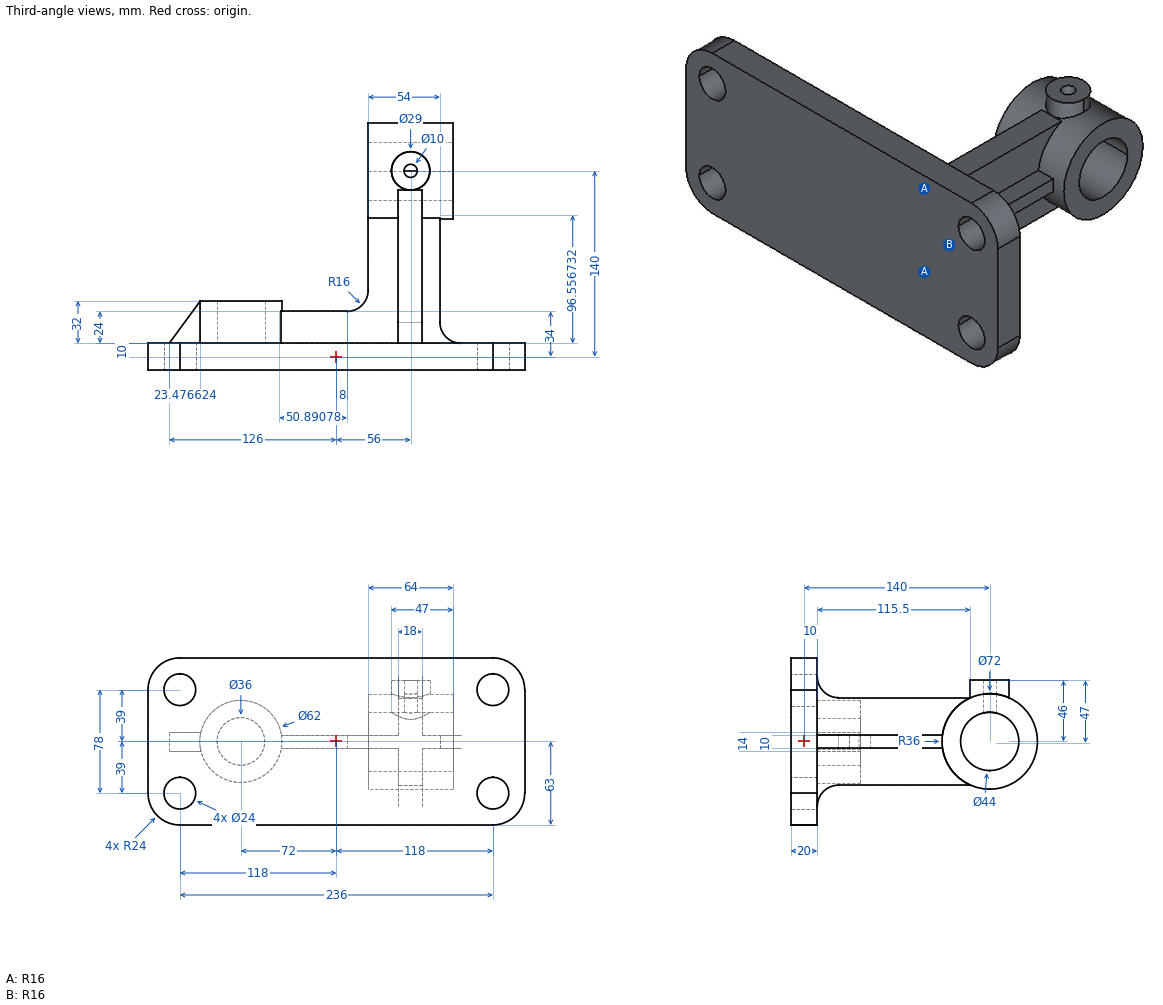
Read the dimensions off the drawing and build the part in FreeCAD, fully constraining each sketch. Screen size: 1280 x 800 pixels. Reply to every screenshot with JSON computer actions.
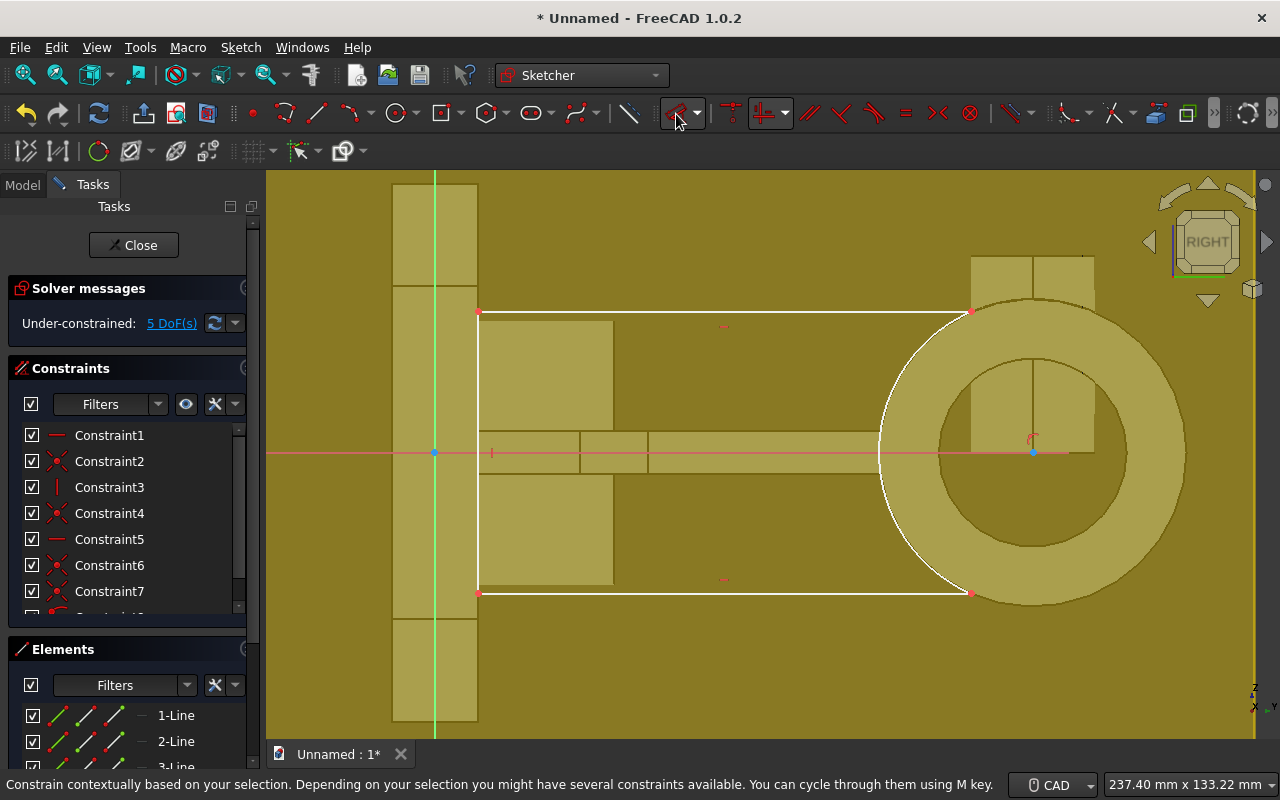
{"action": "left_click", "coordinate": [895, 384]}
{"action": "left_click", "coordinate": [866, 370]}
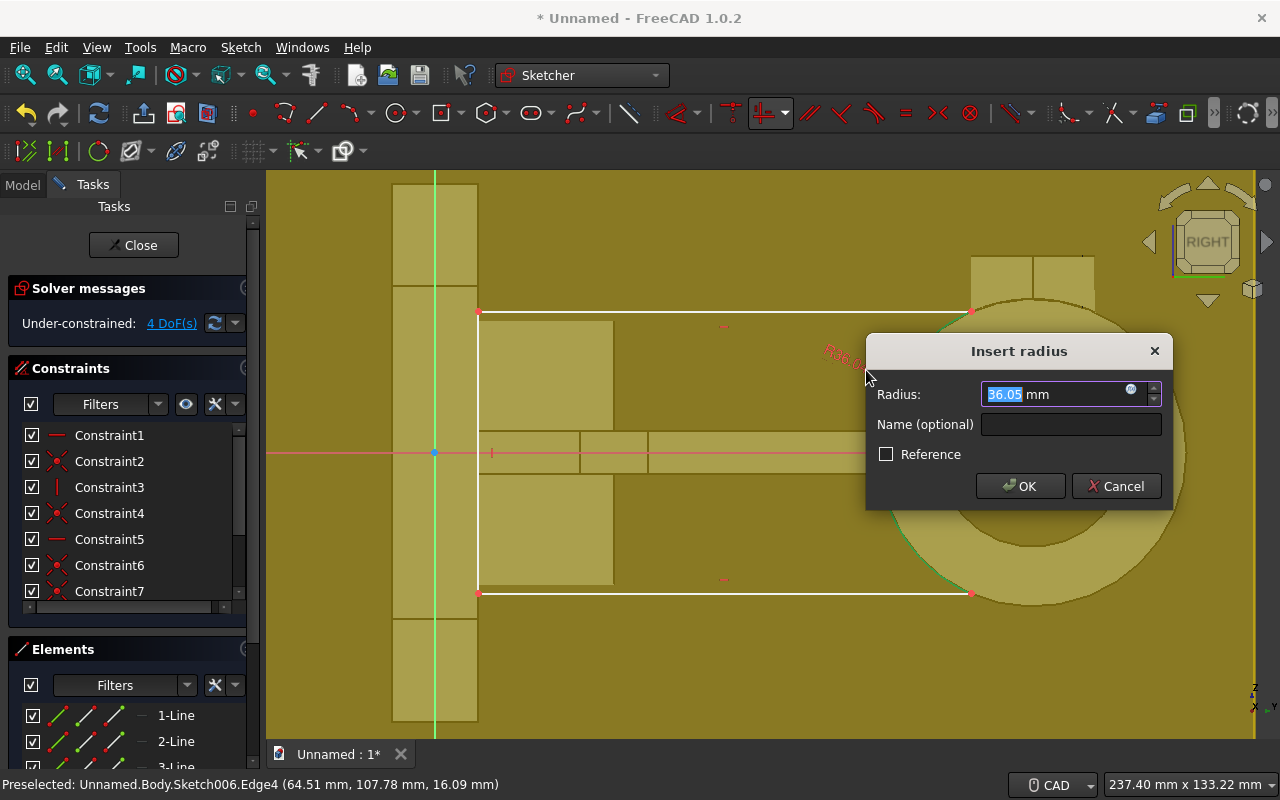
{"action": "type", "text": "36"}
{"action": "key", "text": "Return"}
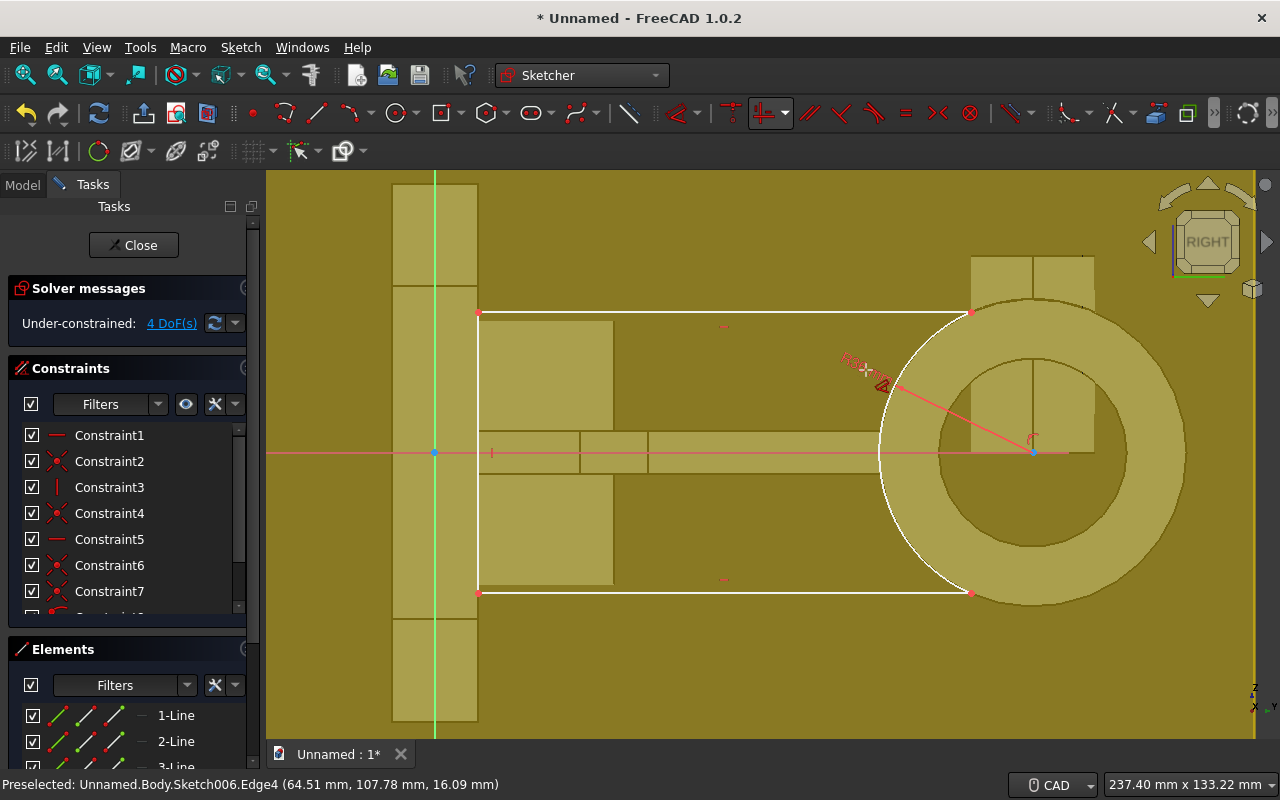
{"action": "left_click", "coordinate": [478, 312]}
{"action": "left_click", "coordinate": [456, 278]}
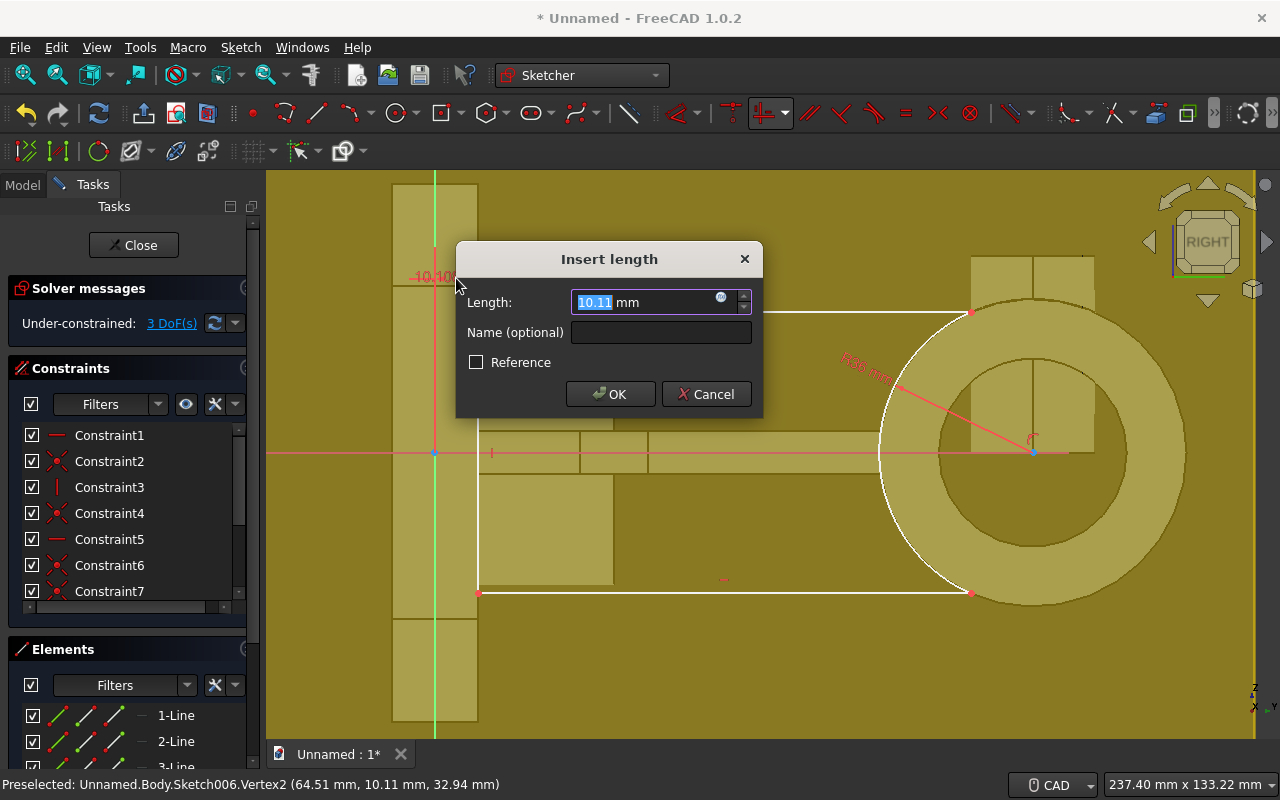
{"action": "type", "text": "10"}
{"action": "key", "text": "Return"}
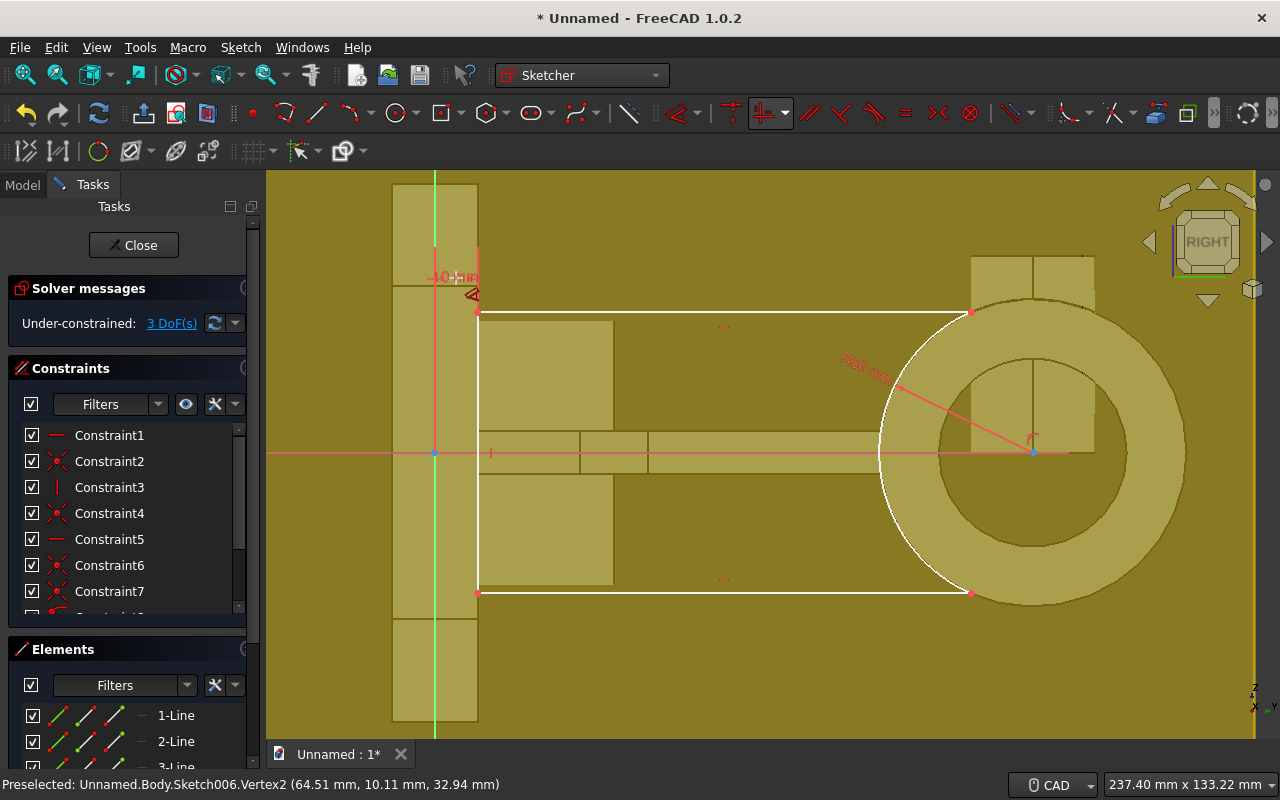
{"action": "left_click", "coordinate": [1033, 453]}
{"action": "left_click", "coordinate": [734, 487]}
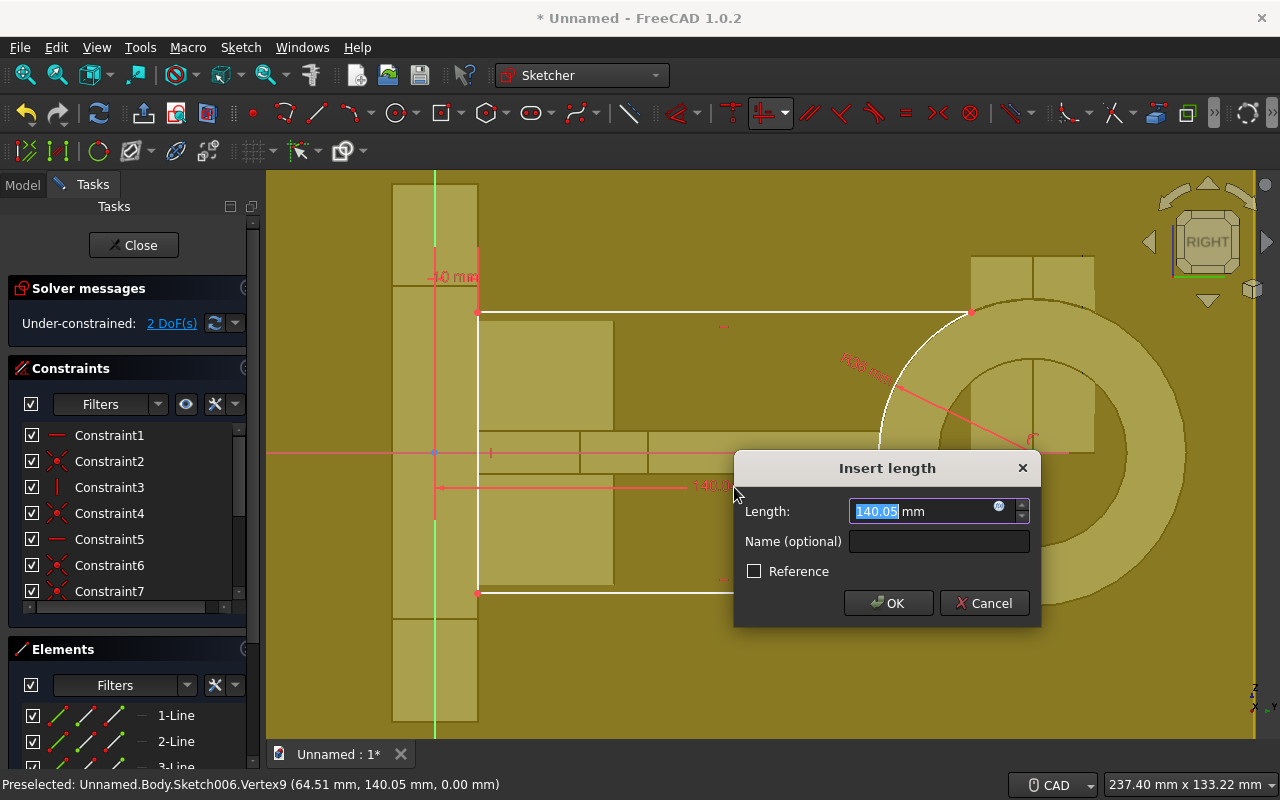
{"action": "type", "text": "140"}
{"action": "key", "text": "Return"}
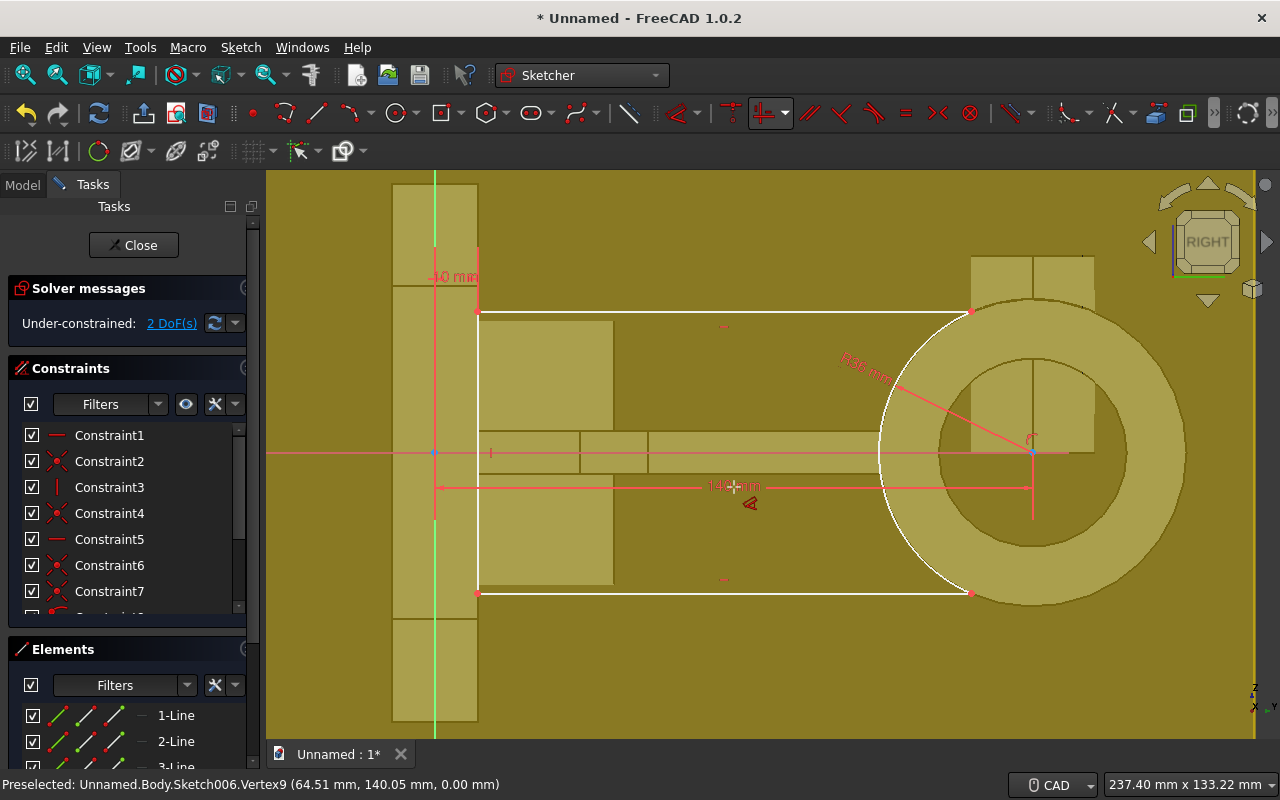
{"action": "left_click", "coordinate": [823, 312]}
{"action": "left_click", "coordinate": [724, 278]}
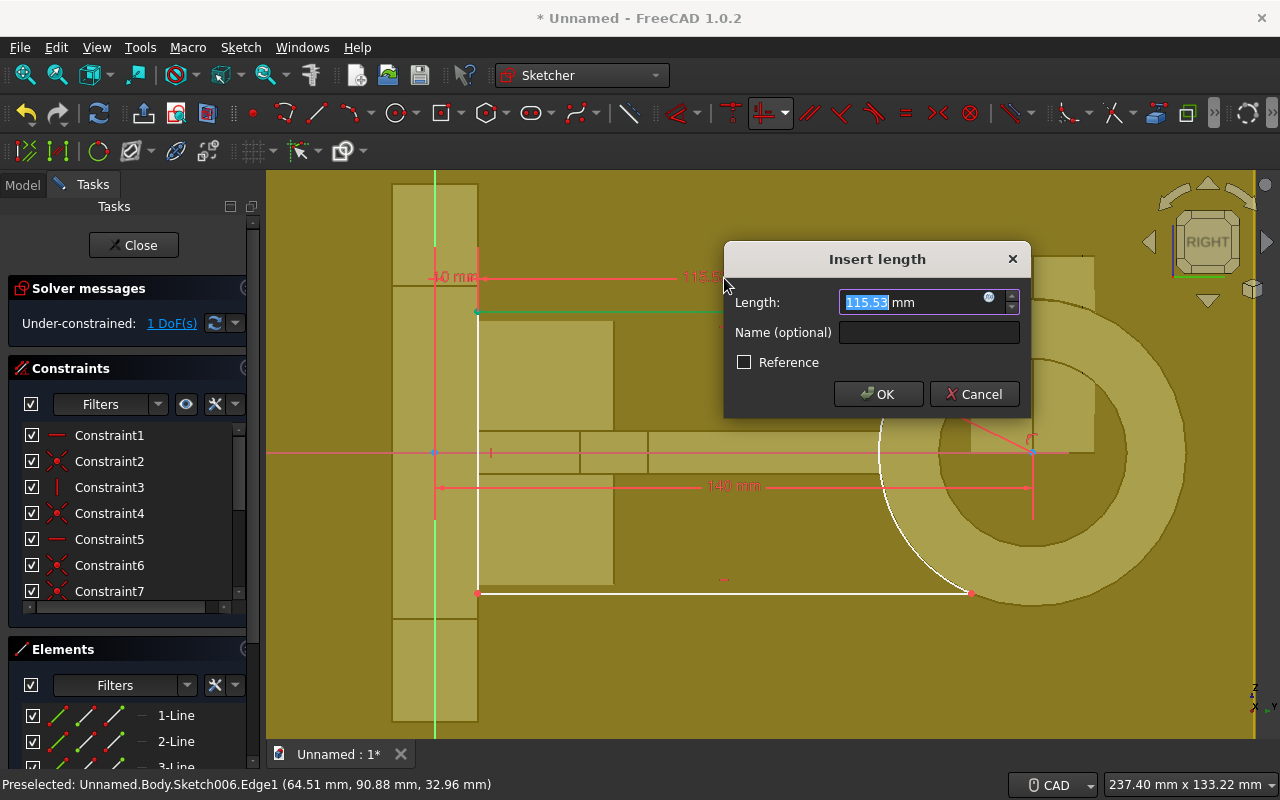
{"action": "type", "text": "115.5"}
{"action": "key", "text": "Return"}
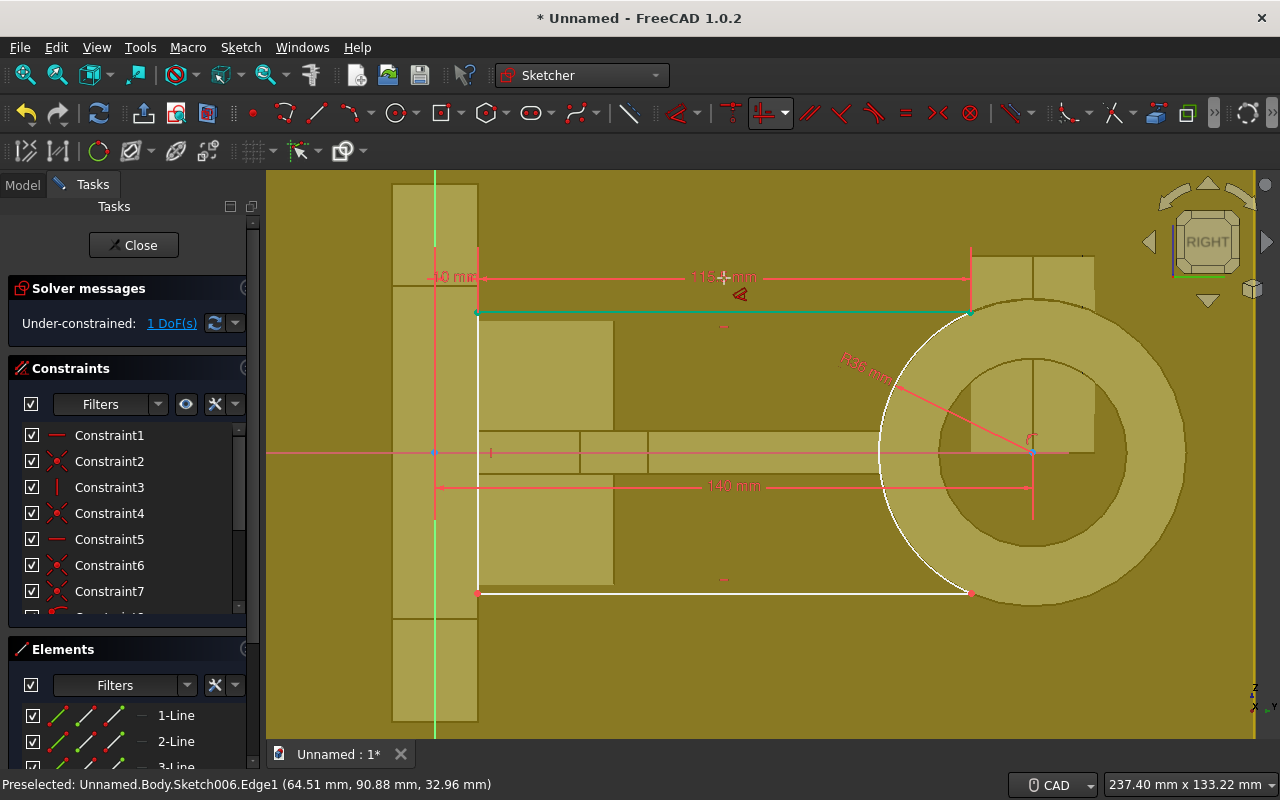
{"action": "left_click", "coordinate": [626, 594]}
{"action": "left_click", "coordinate": [724, 628]}